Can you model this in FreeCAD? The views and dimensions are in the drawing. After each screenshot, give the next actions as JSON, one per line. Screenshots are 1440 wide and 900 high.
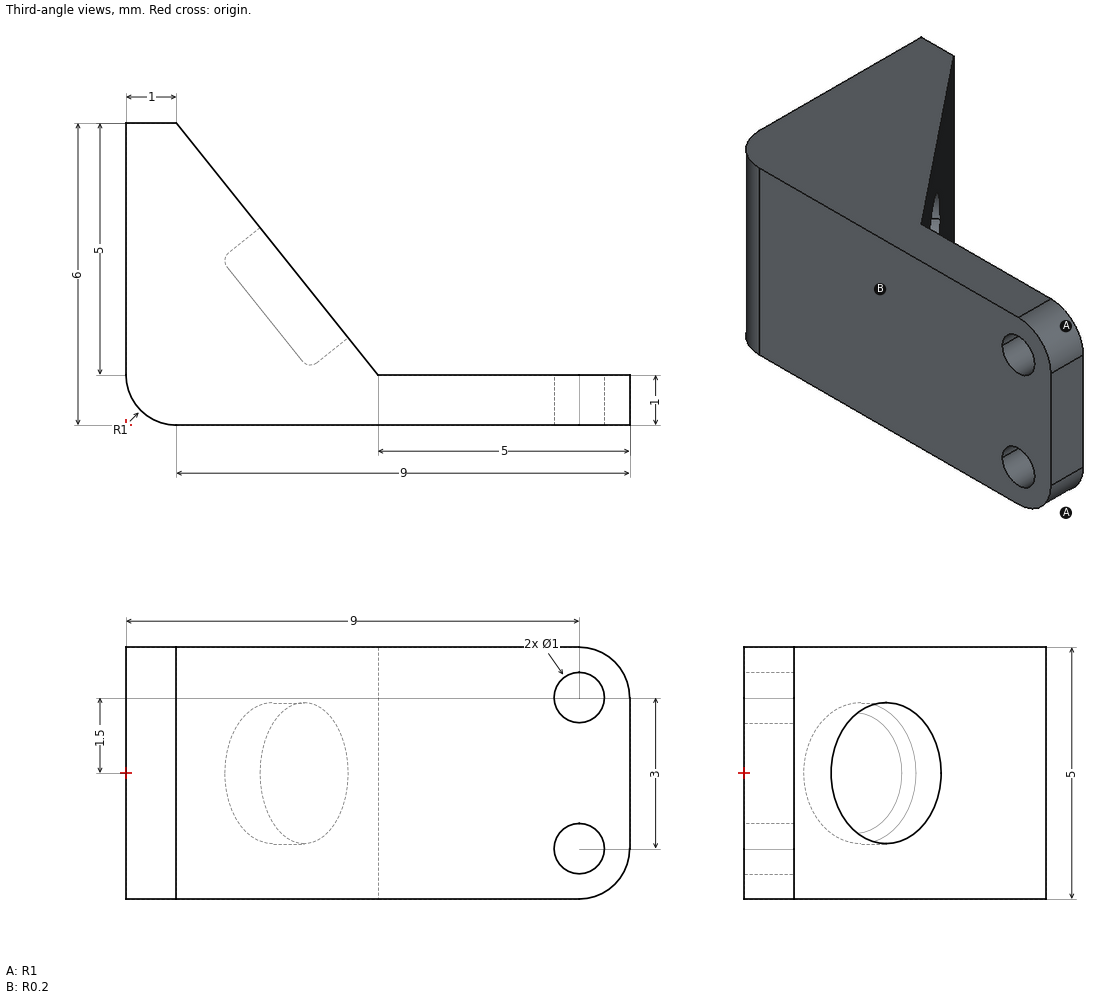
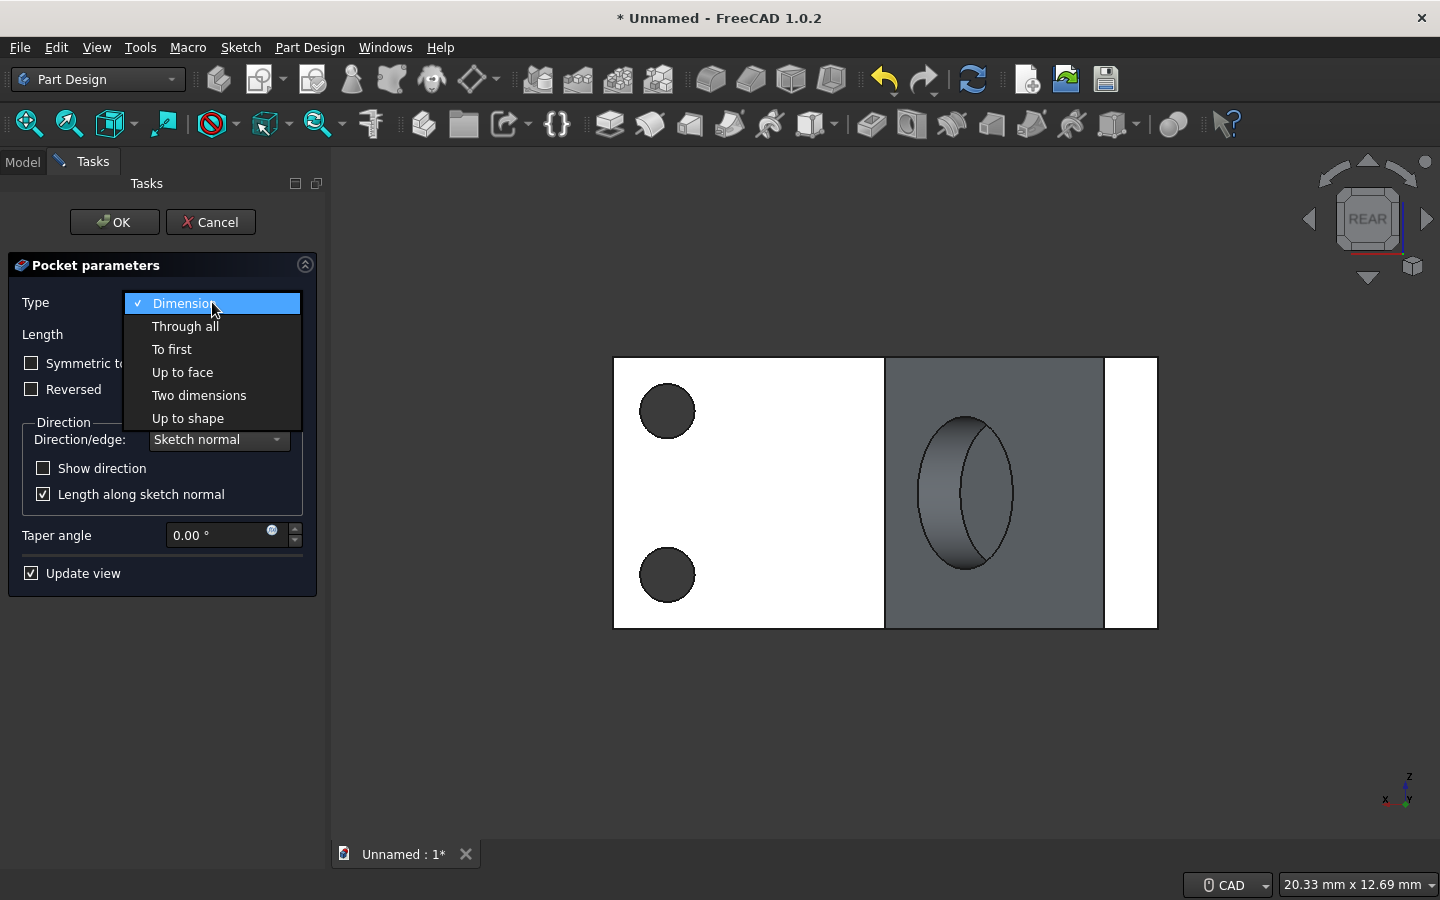
{"action": "left_click", "coordinate": [212, 326]}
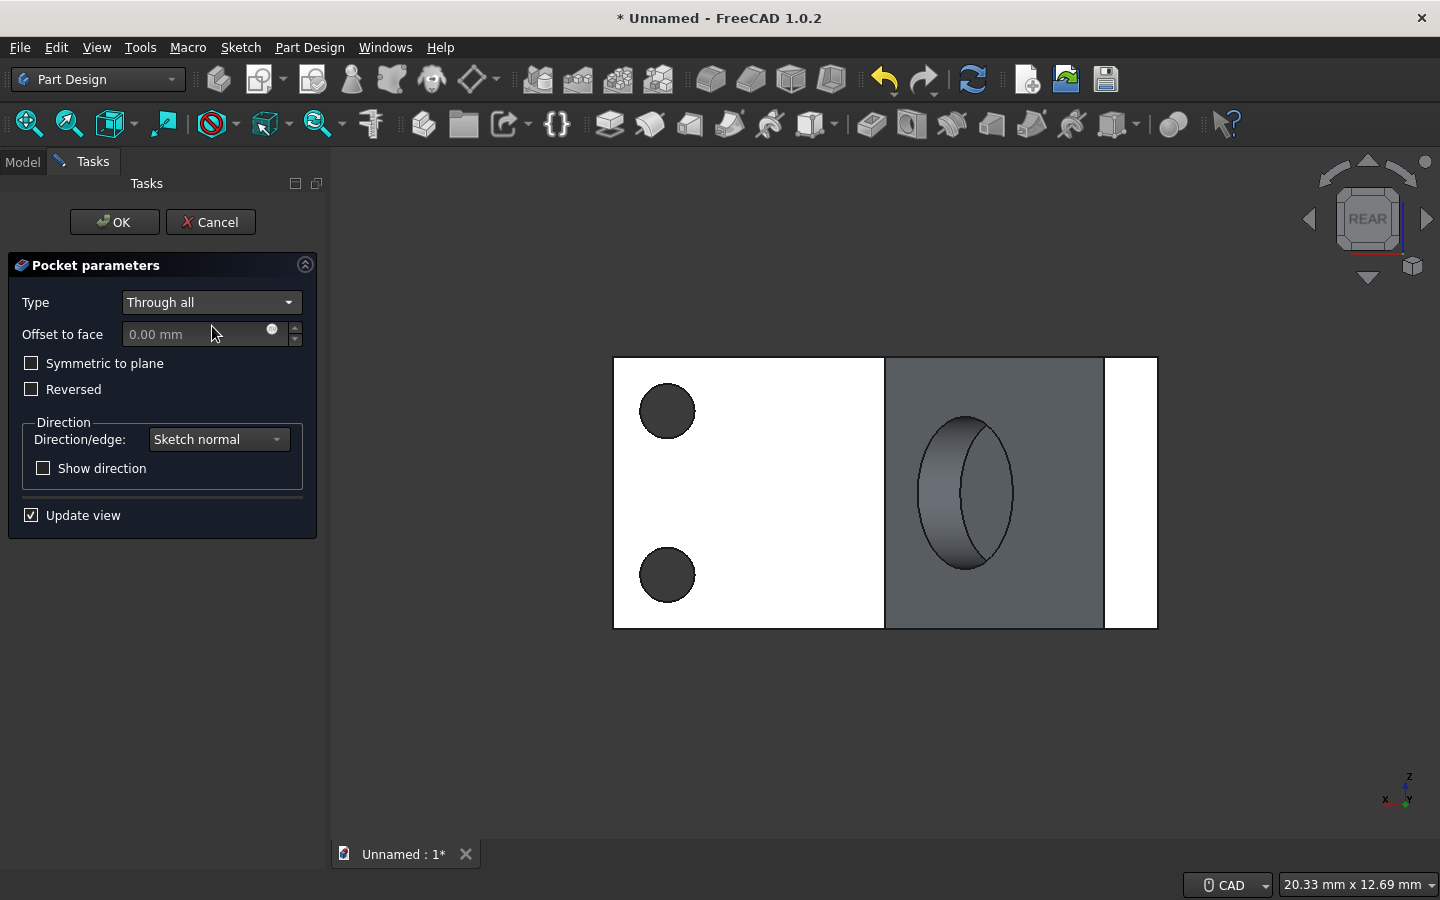
{"action": "left_click", "coordinate": [115, 222]}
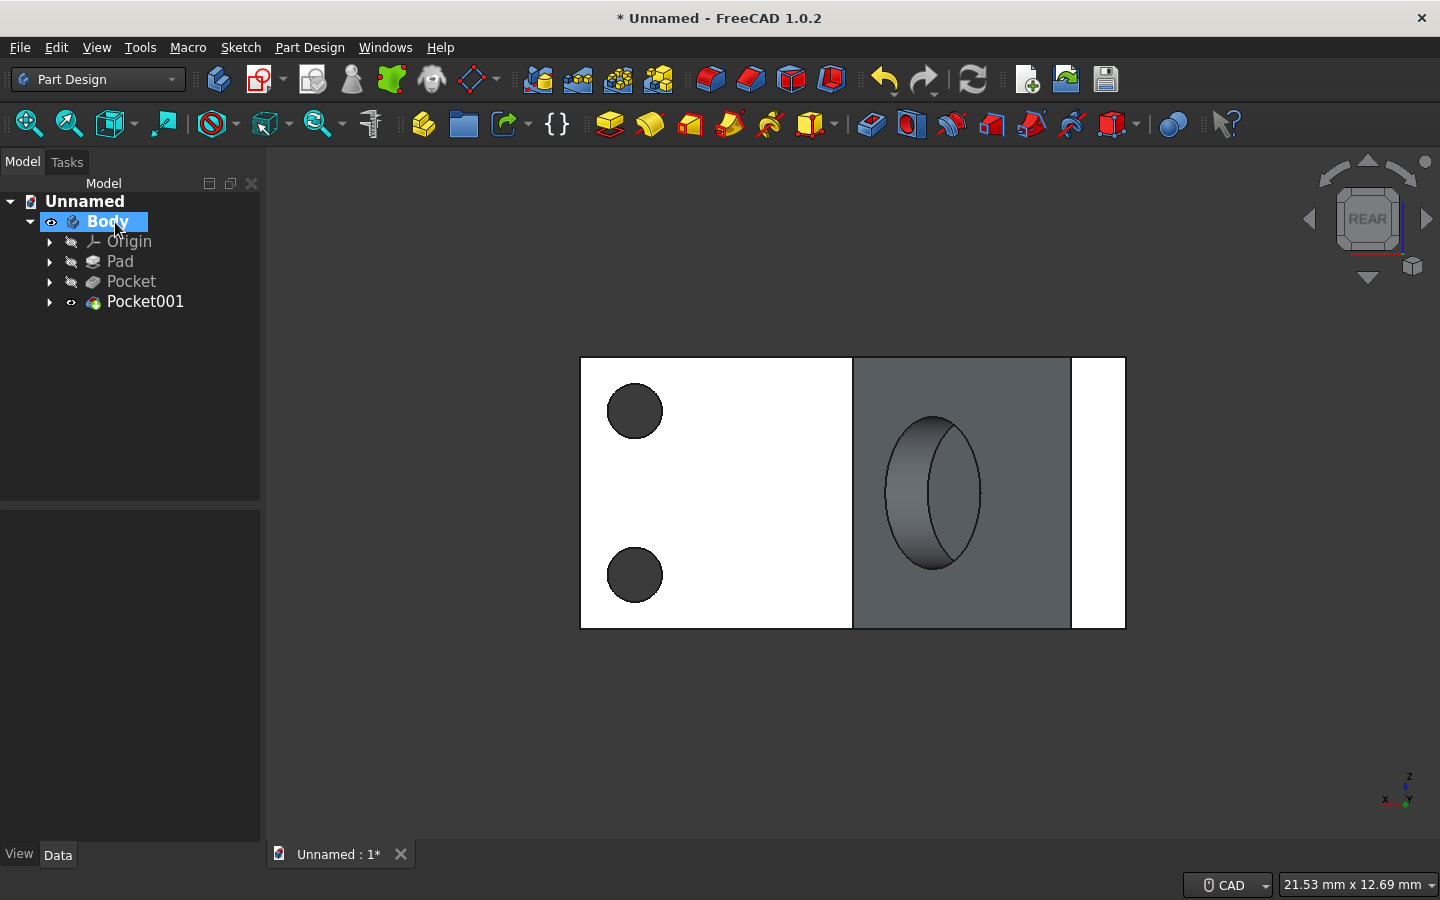
{"action": "key", "text": "0"}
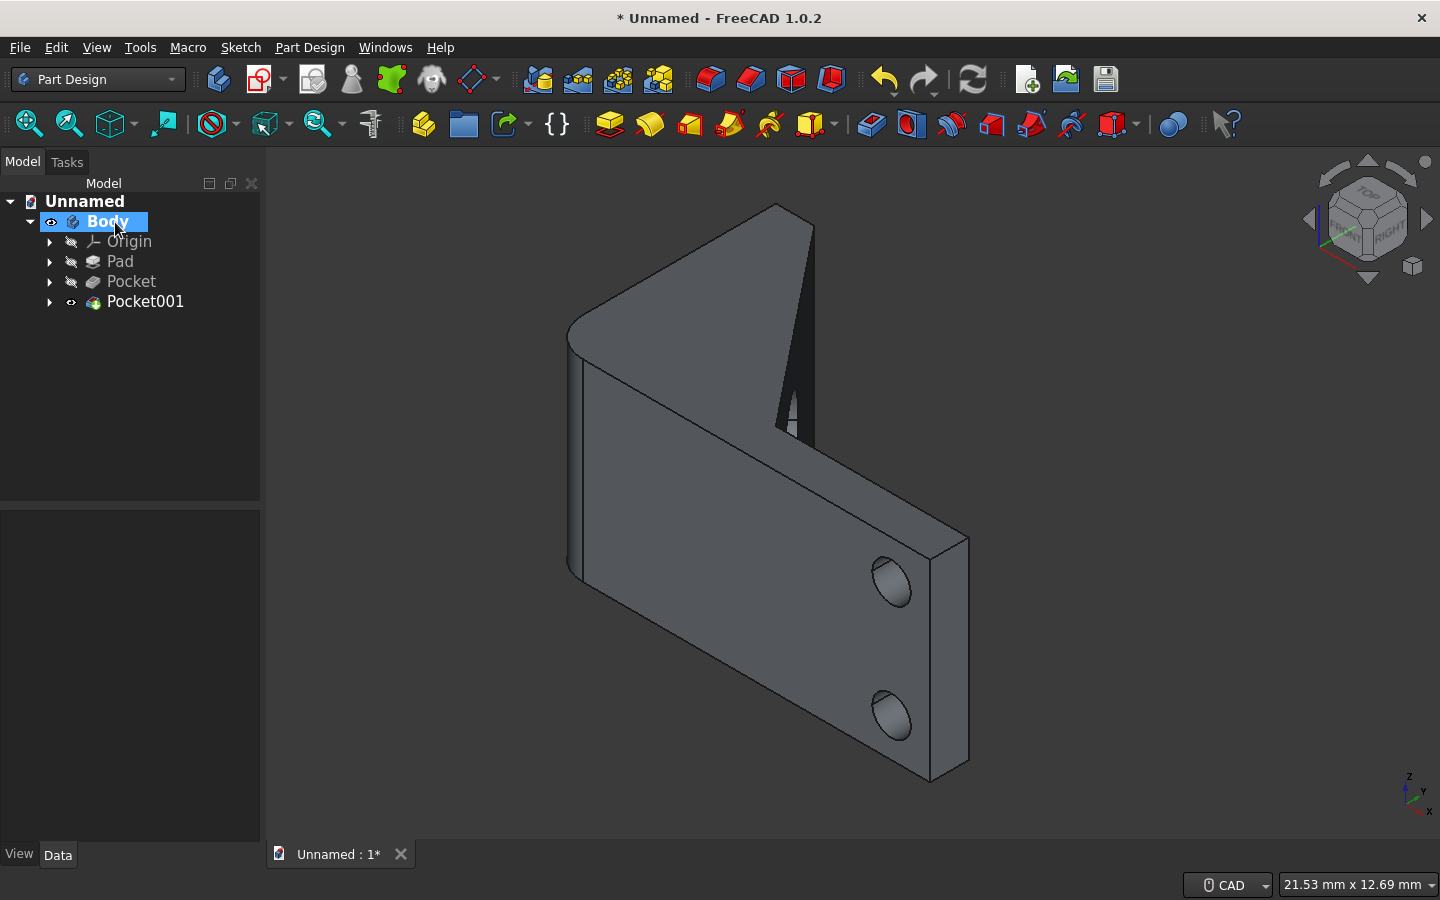
{"action": "left_click", "coordinate": [949, 548]}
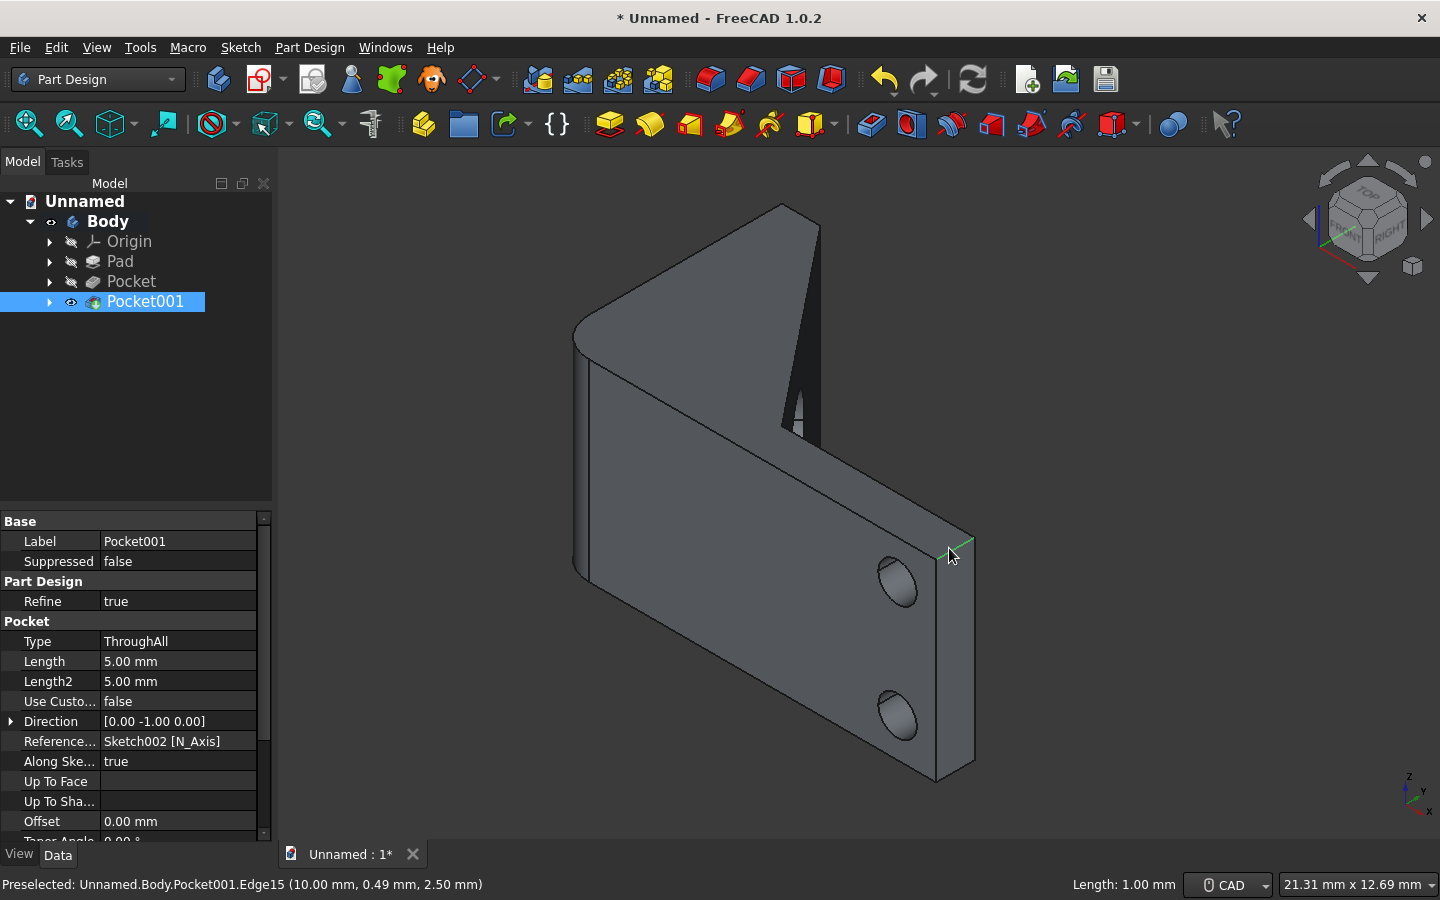
{"action": "key", "text": "2"}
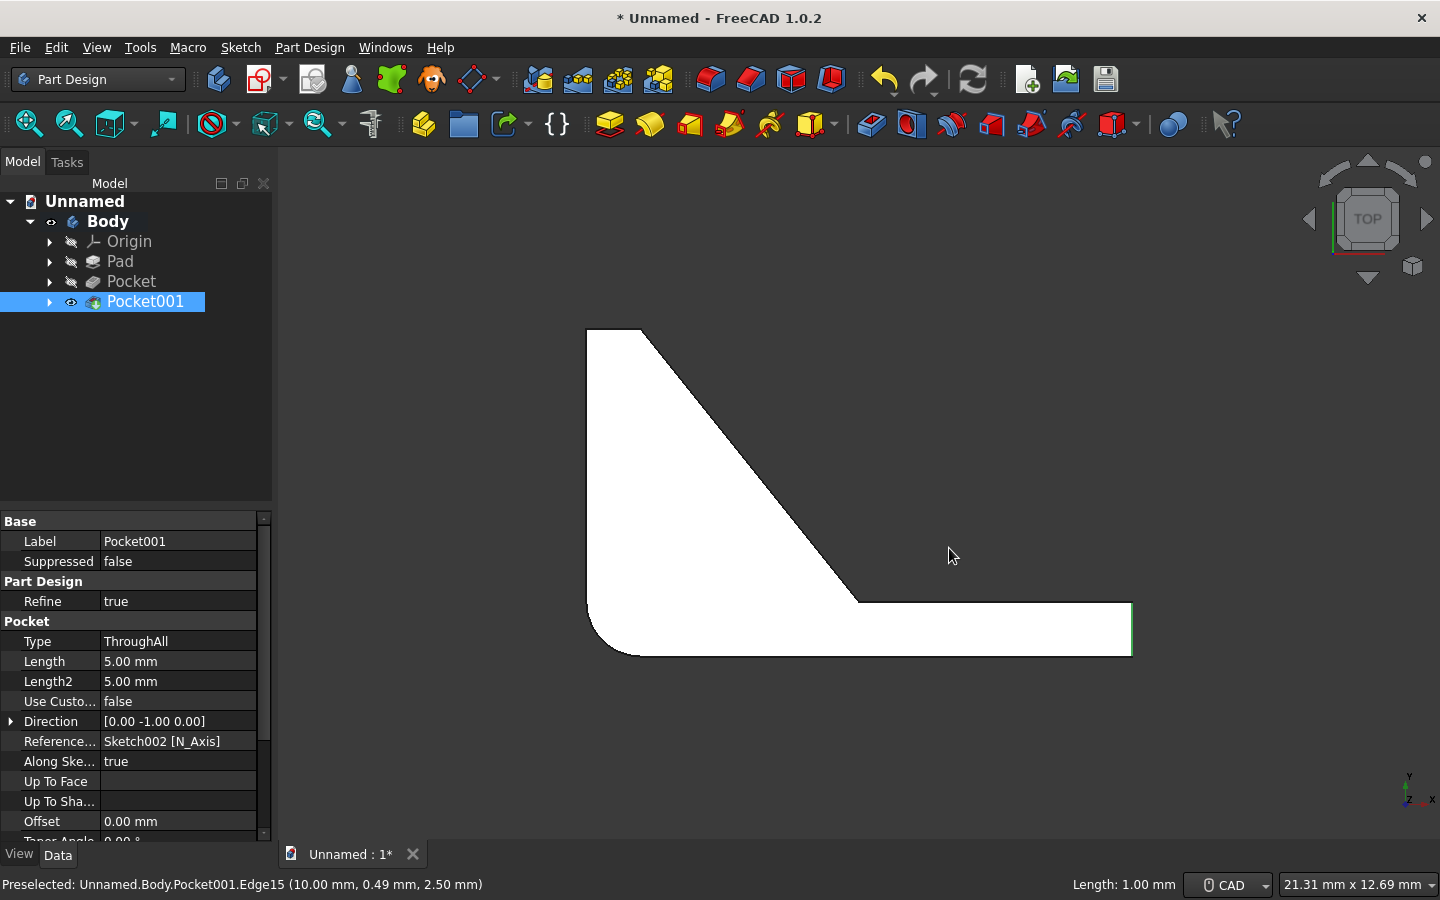
{"action": "key", "text": "1"}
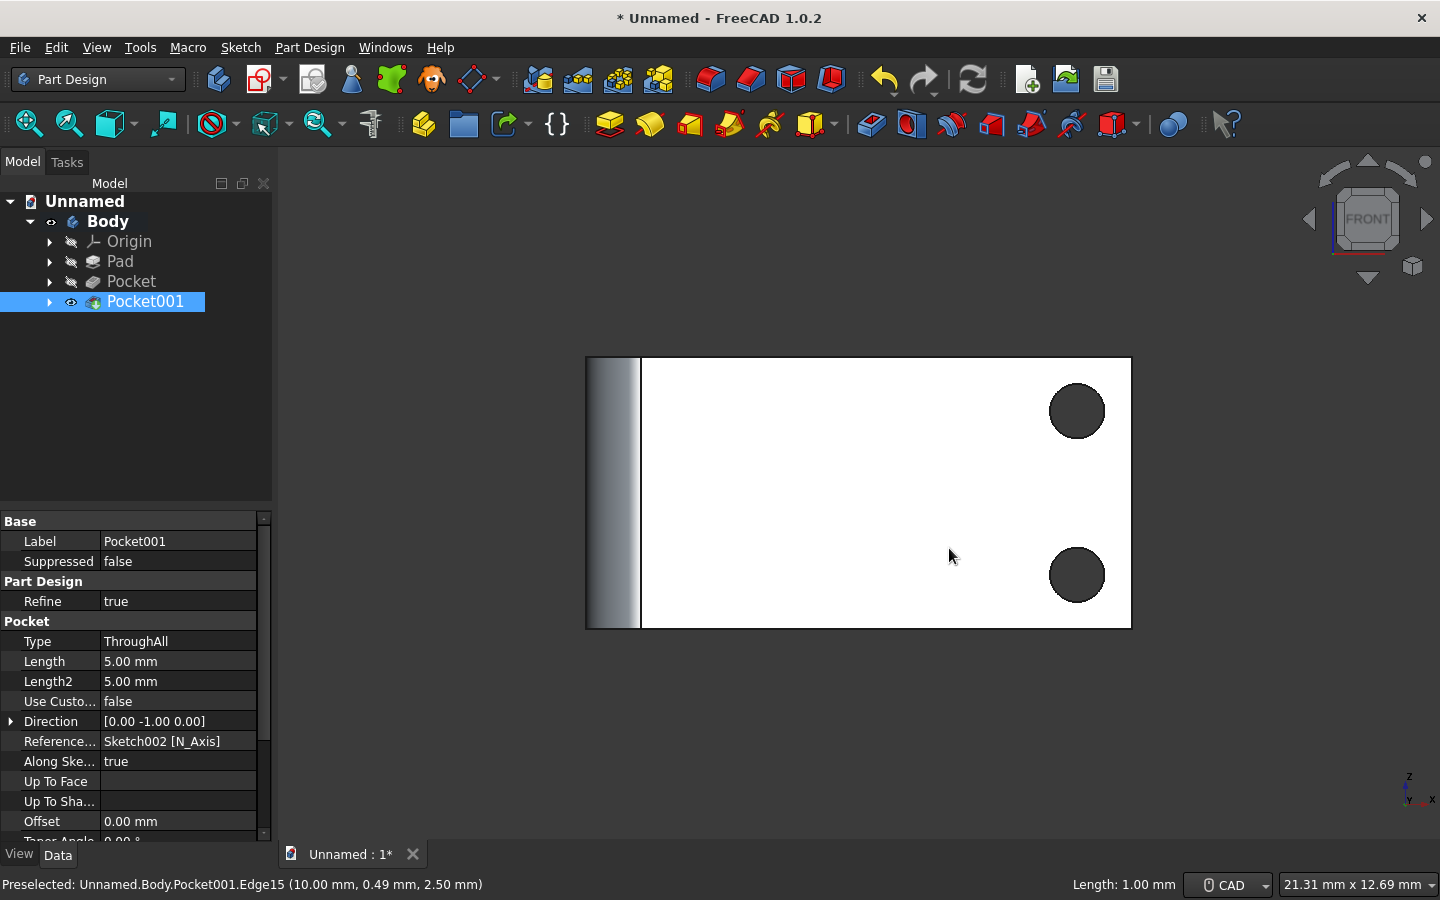
{"action": "key", "text": "3"}